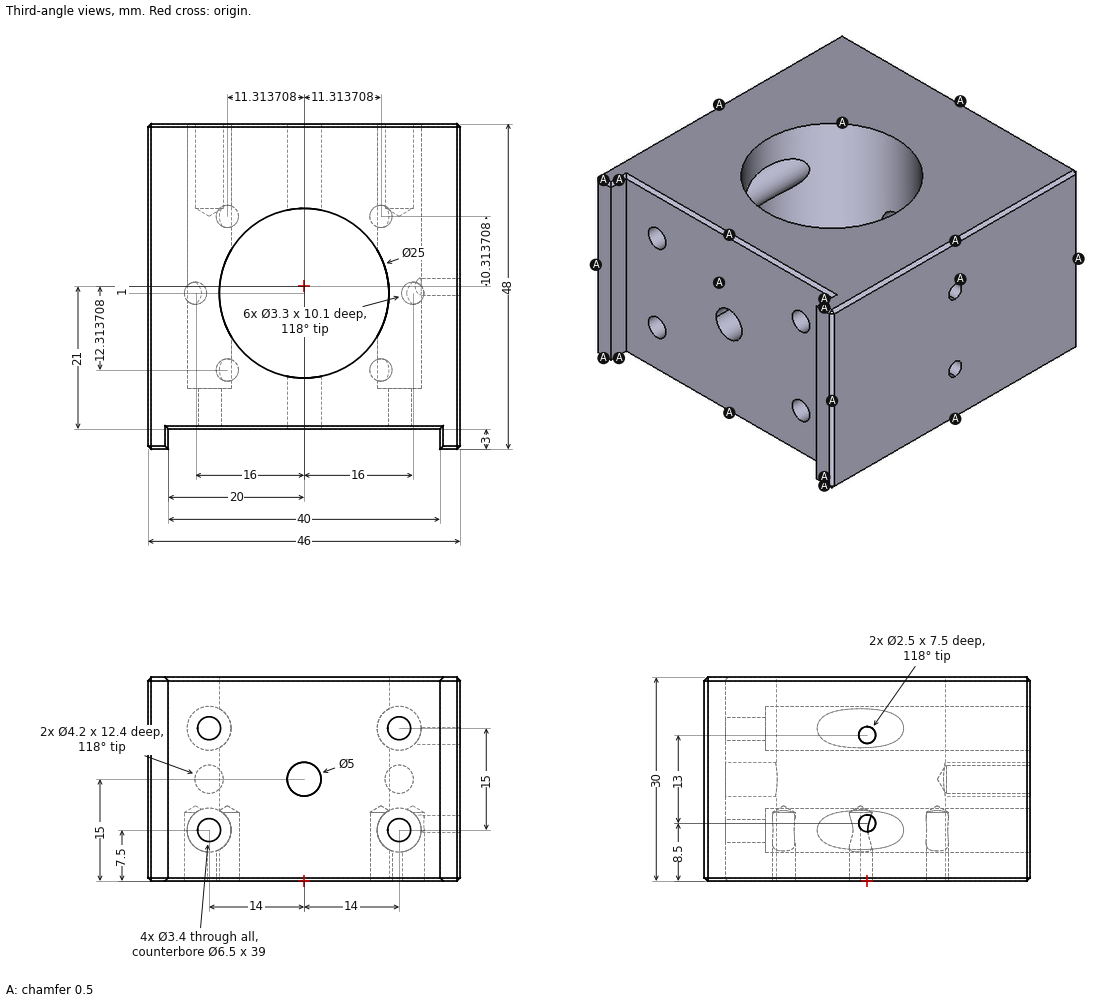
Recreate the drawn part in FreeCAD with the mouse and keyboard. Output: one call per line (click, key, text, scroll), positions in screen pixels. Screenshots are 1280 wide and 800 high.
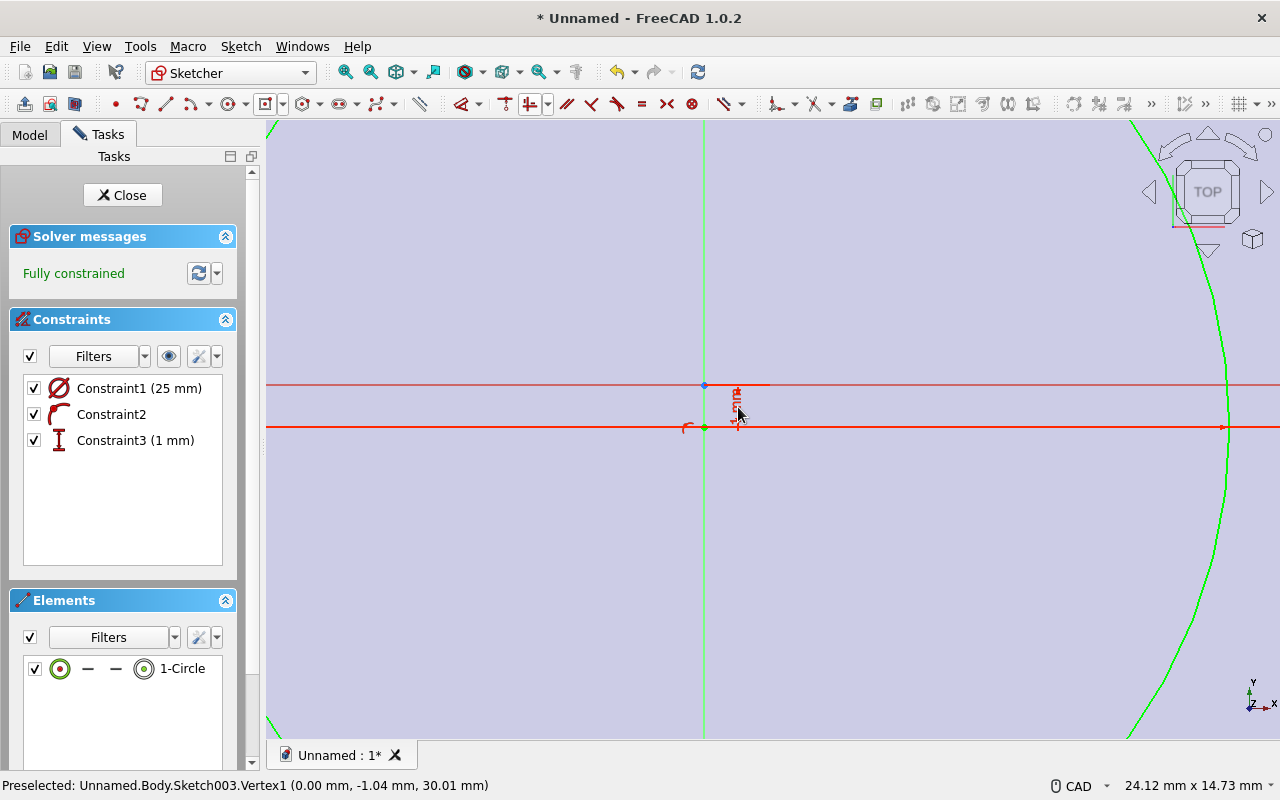
click(123, 195)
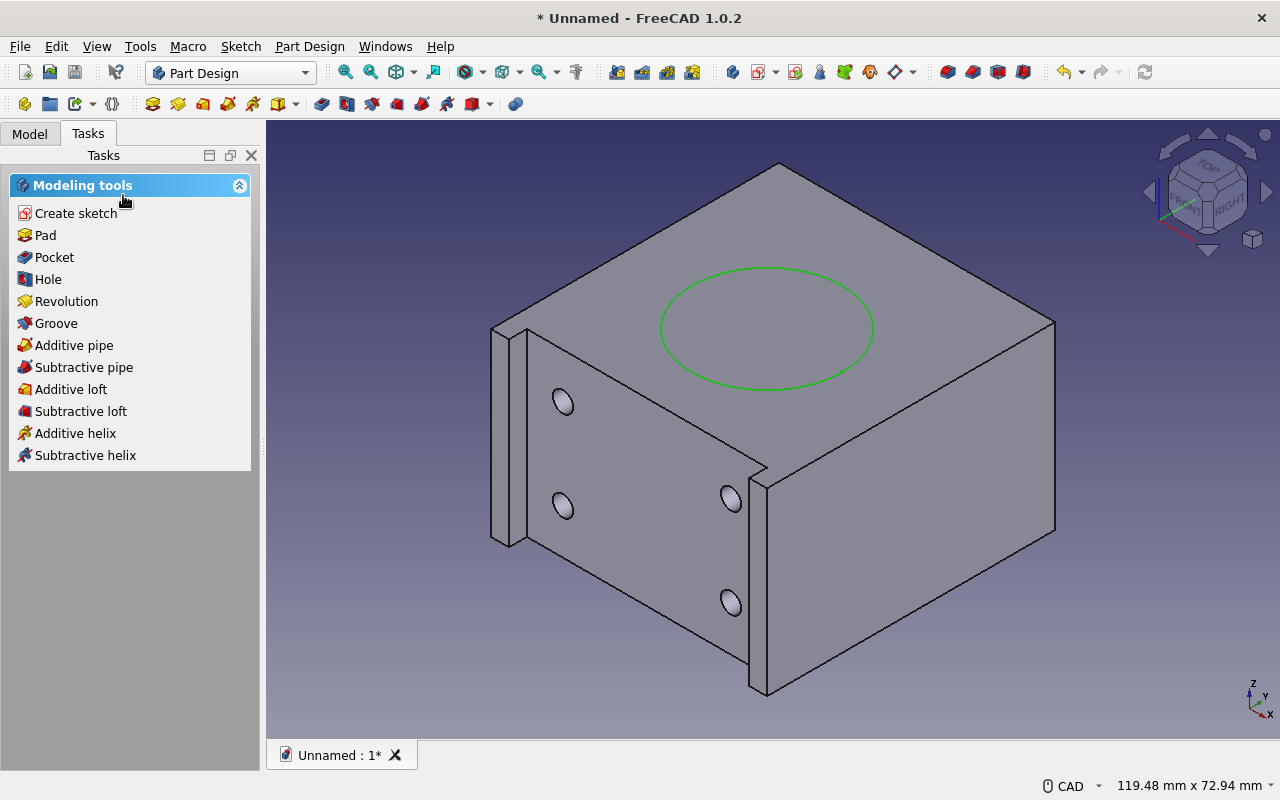
click(322, 104)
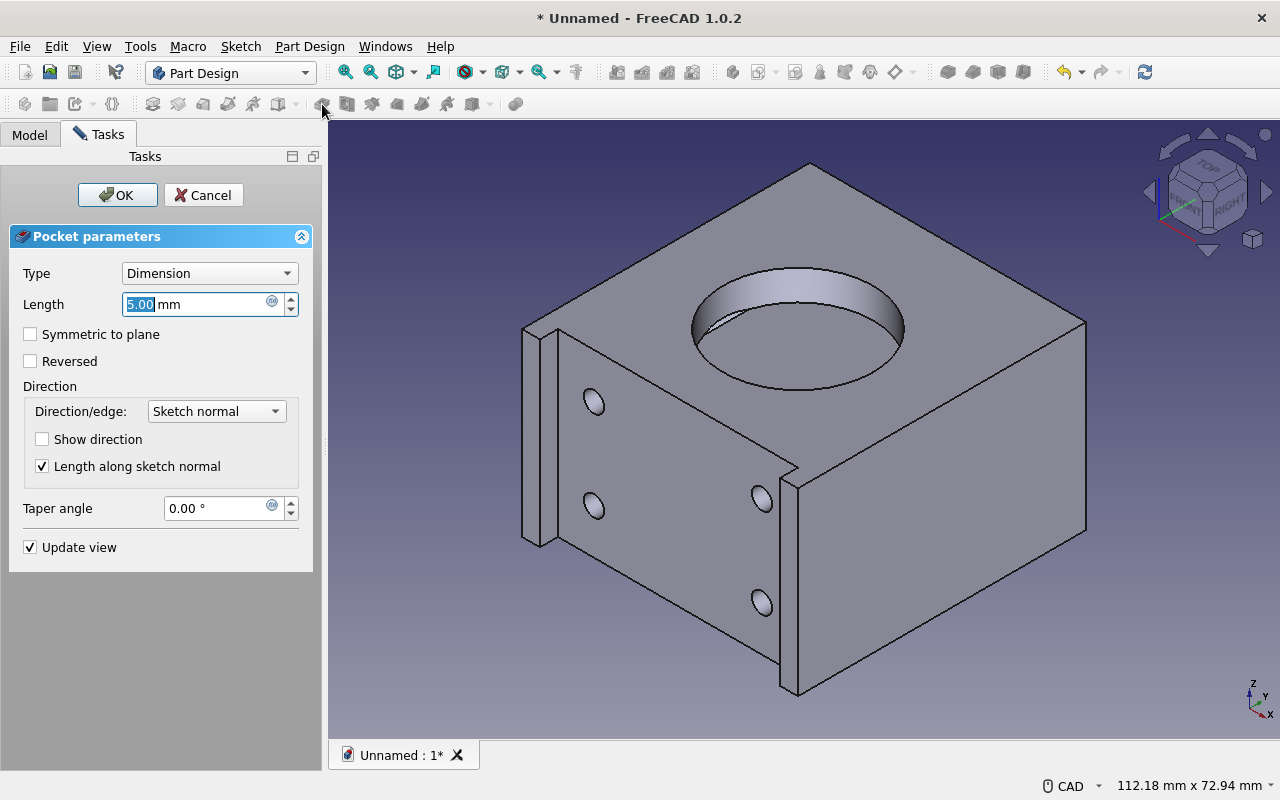
click(210, 274)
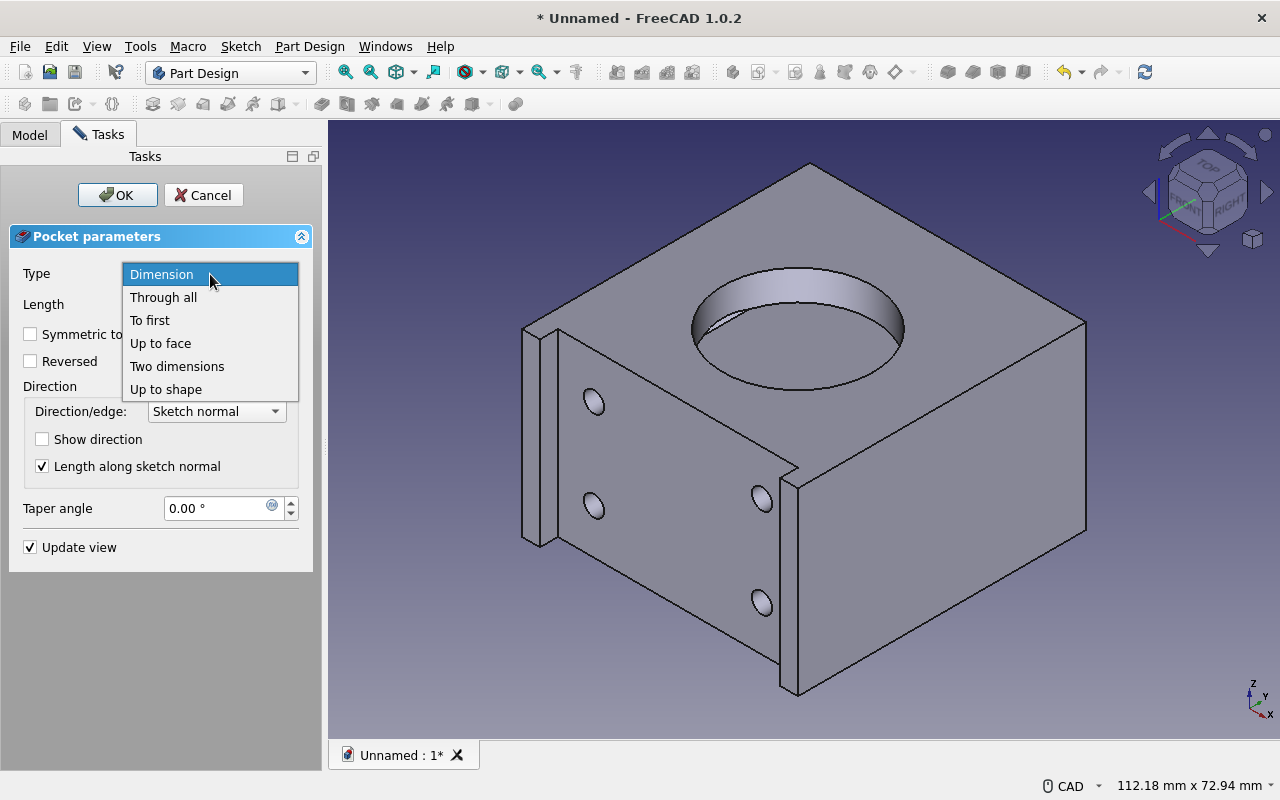
click(208, 298)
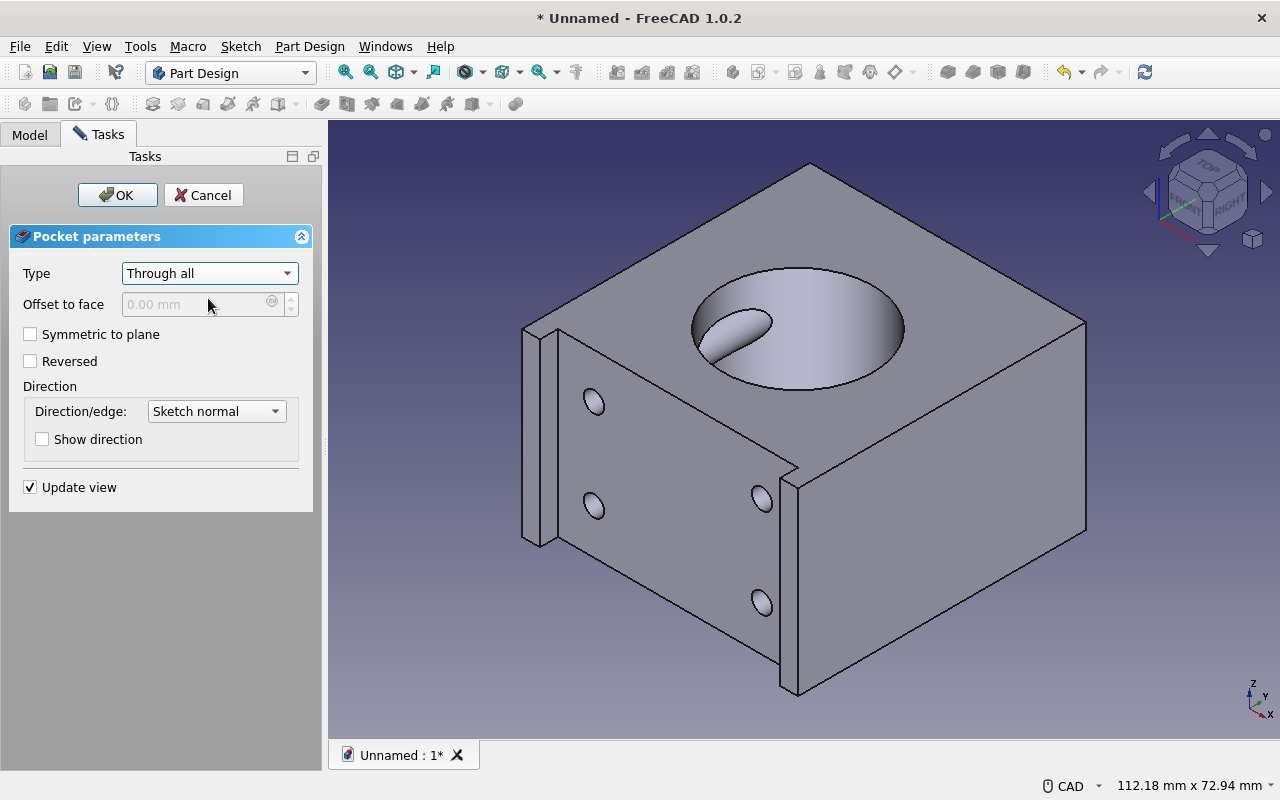
click(118, 195)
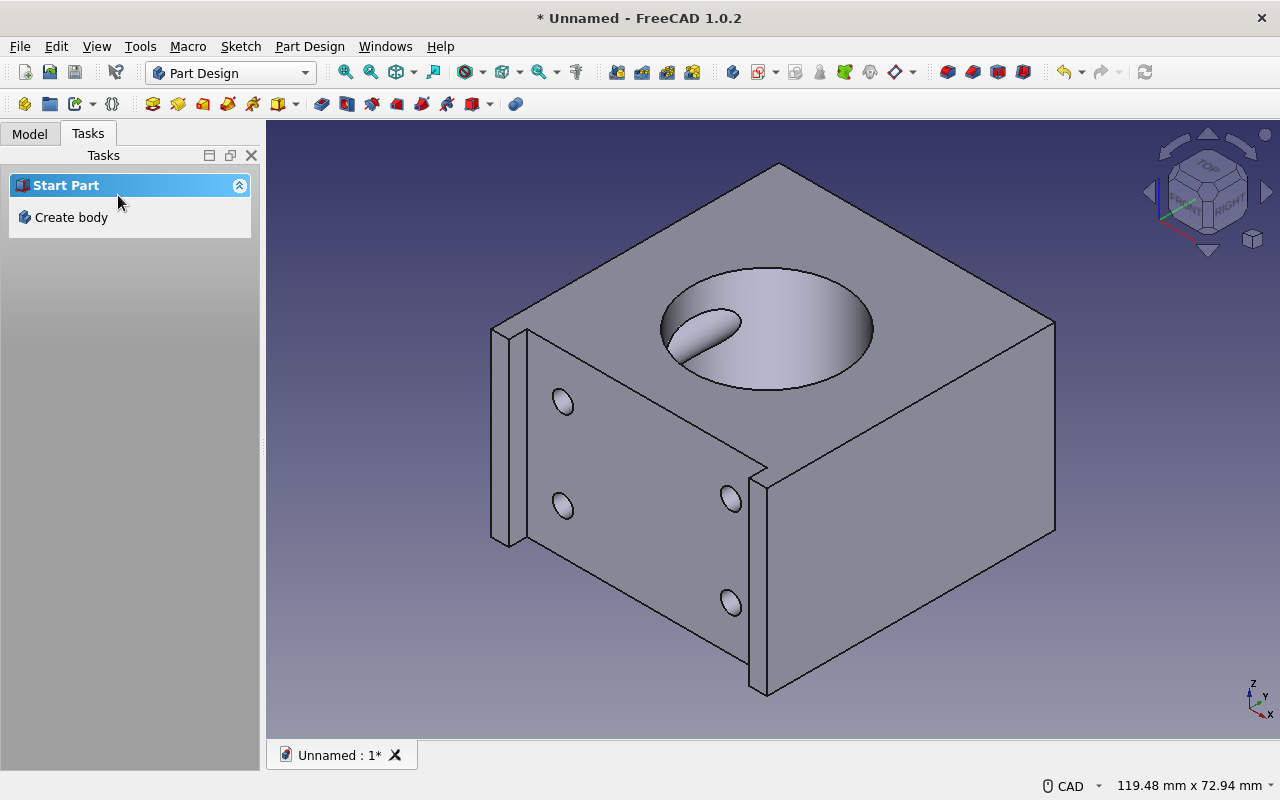
key(4)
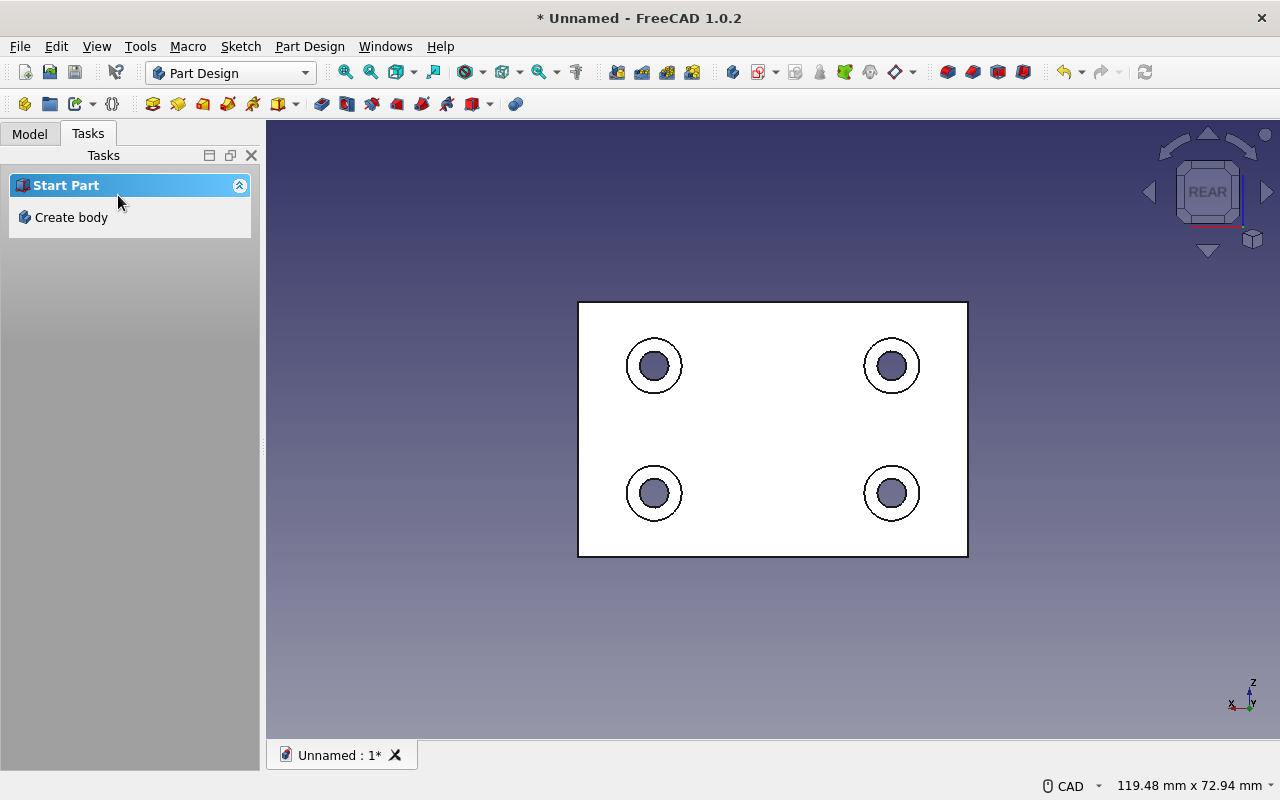
click(346, 72)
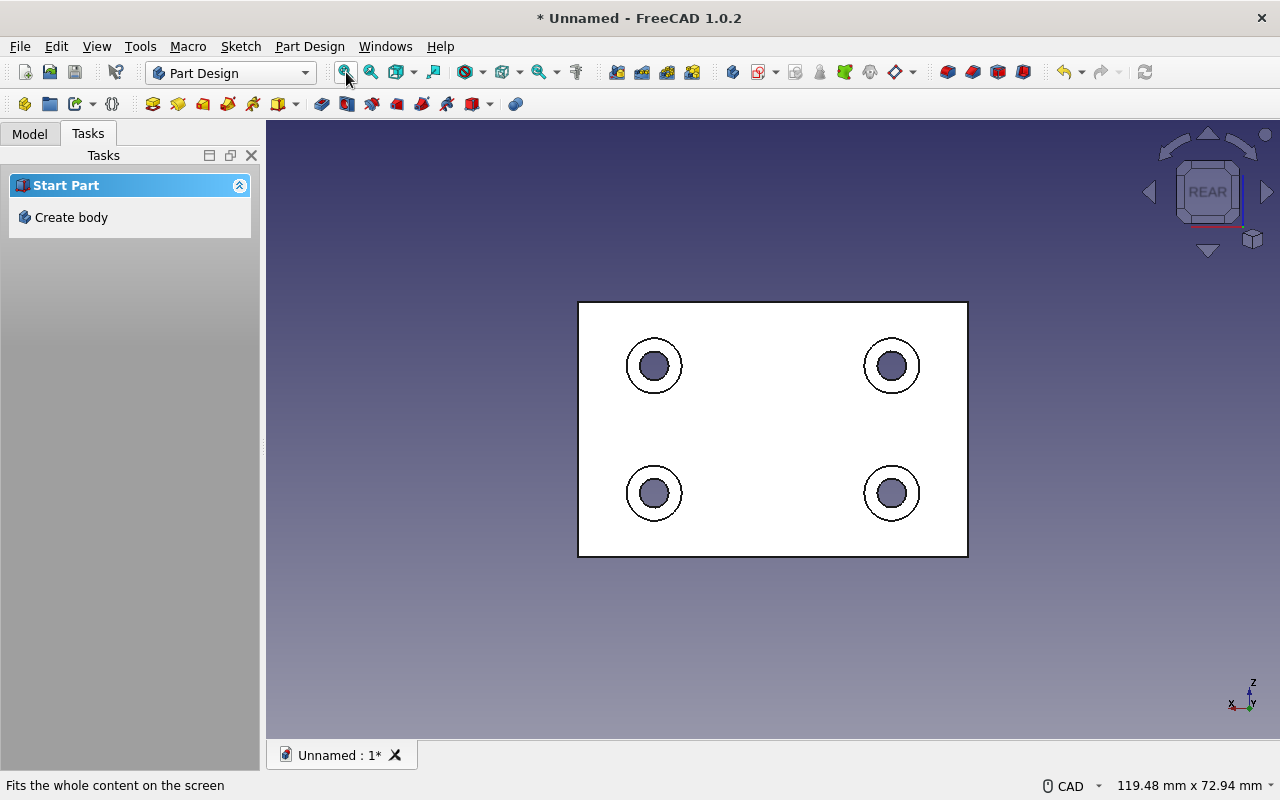
click(773, 429)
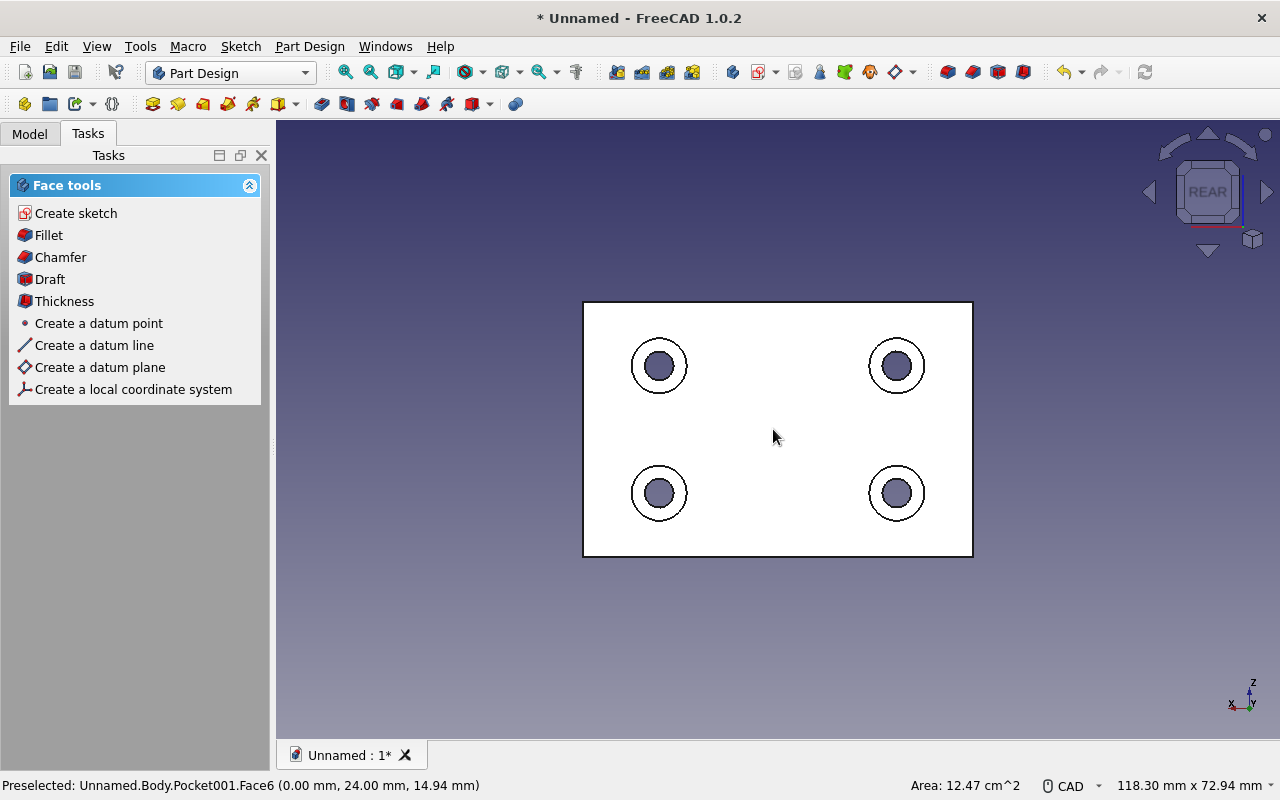
click(758, 72)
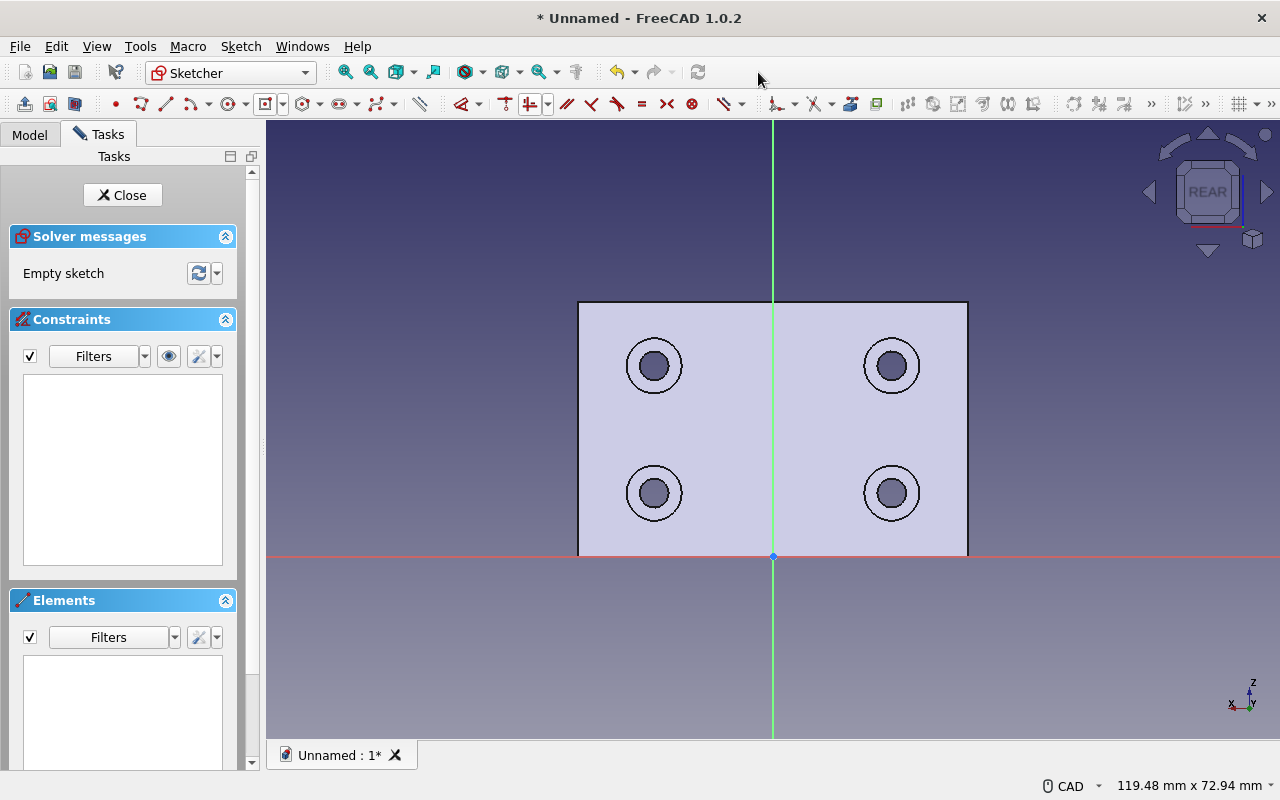
scroll(782, 430, up, 11)